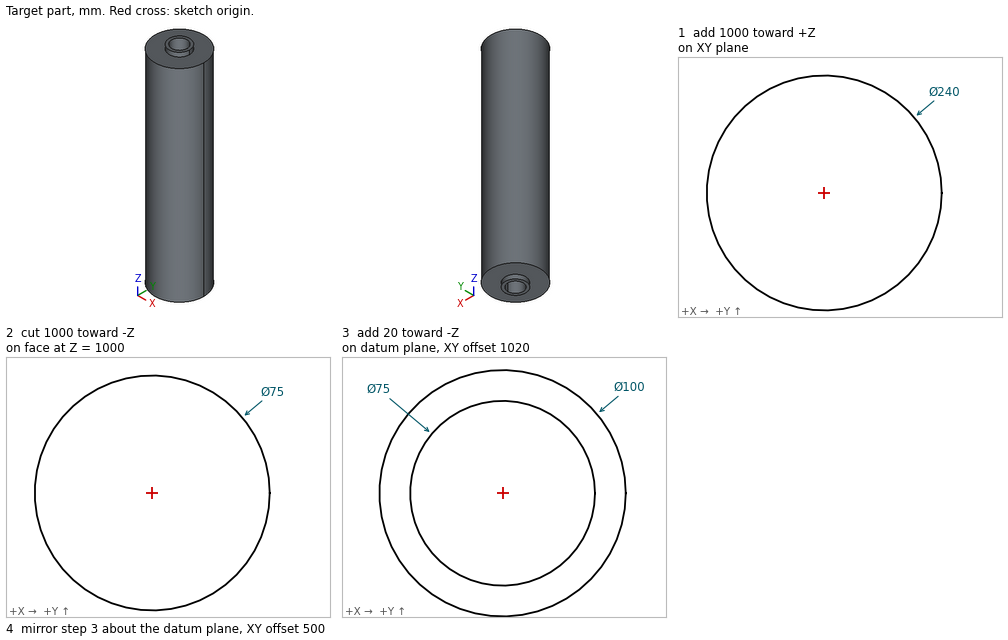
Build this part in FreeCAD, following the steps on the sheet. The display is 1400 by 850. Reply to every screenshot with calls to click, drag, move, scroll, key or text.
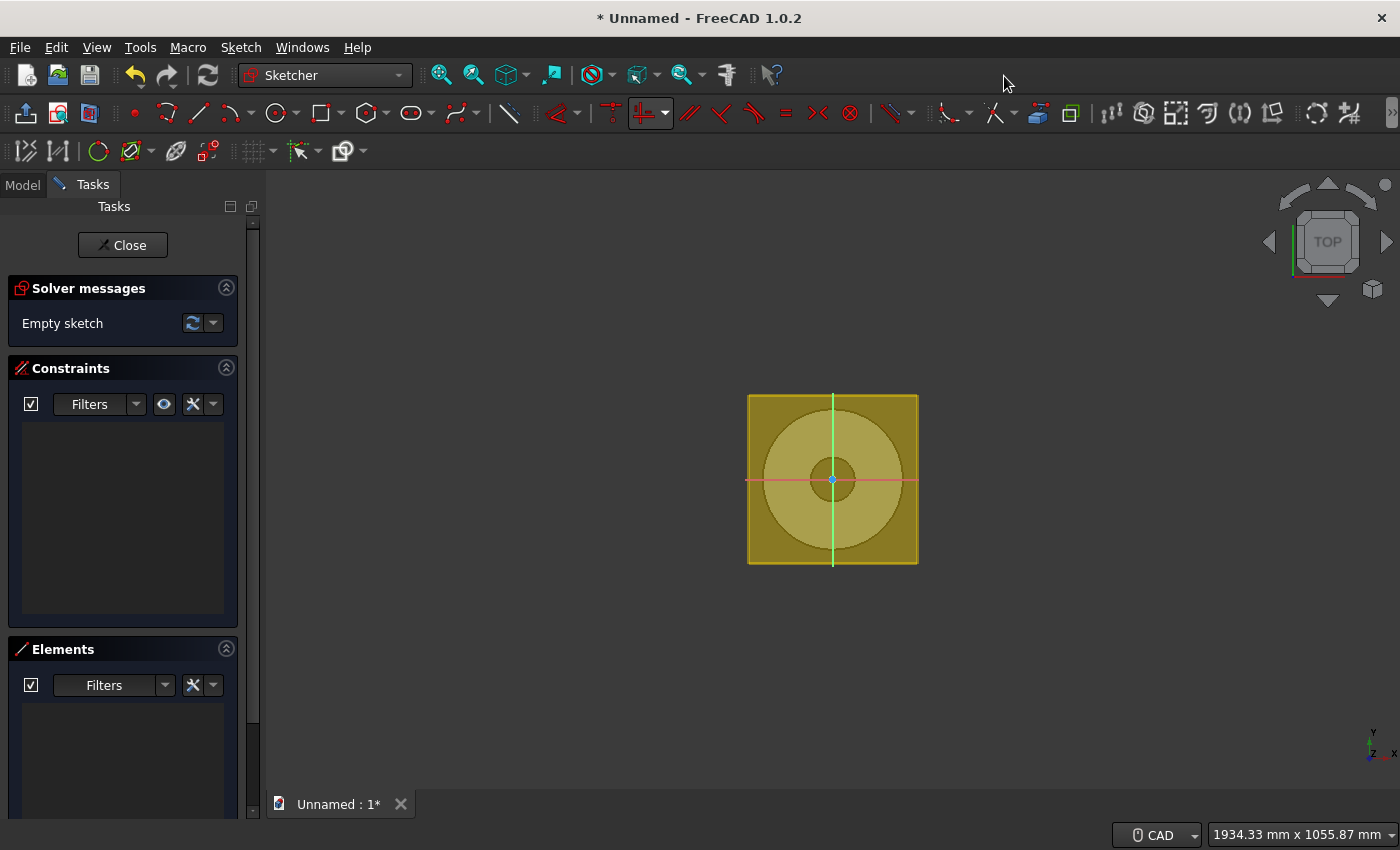
scroll(844, 480, up, 10)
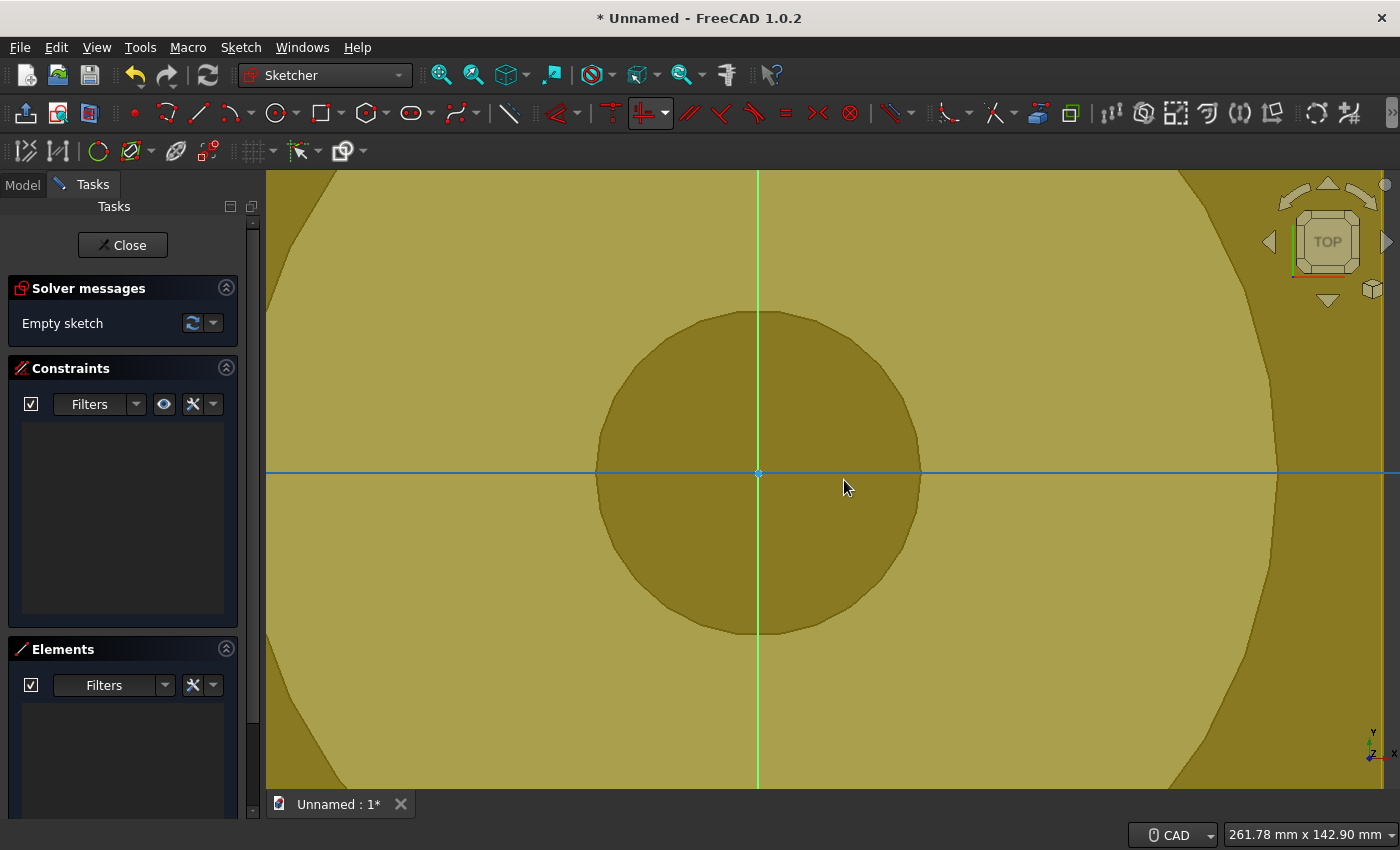
key(g)
key(c)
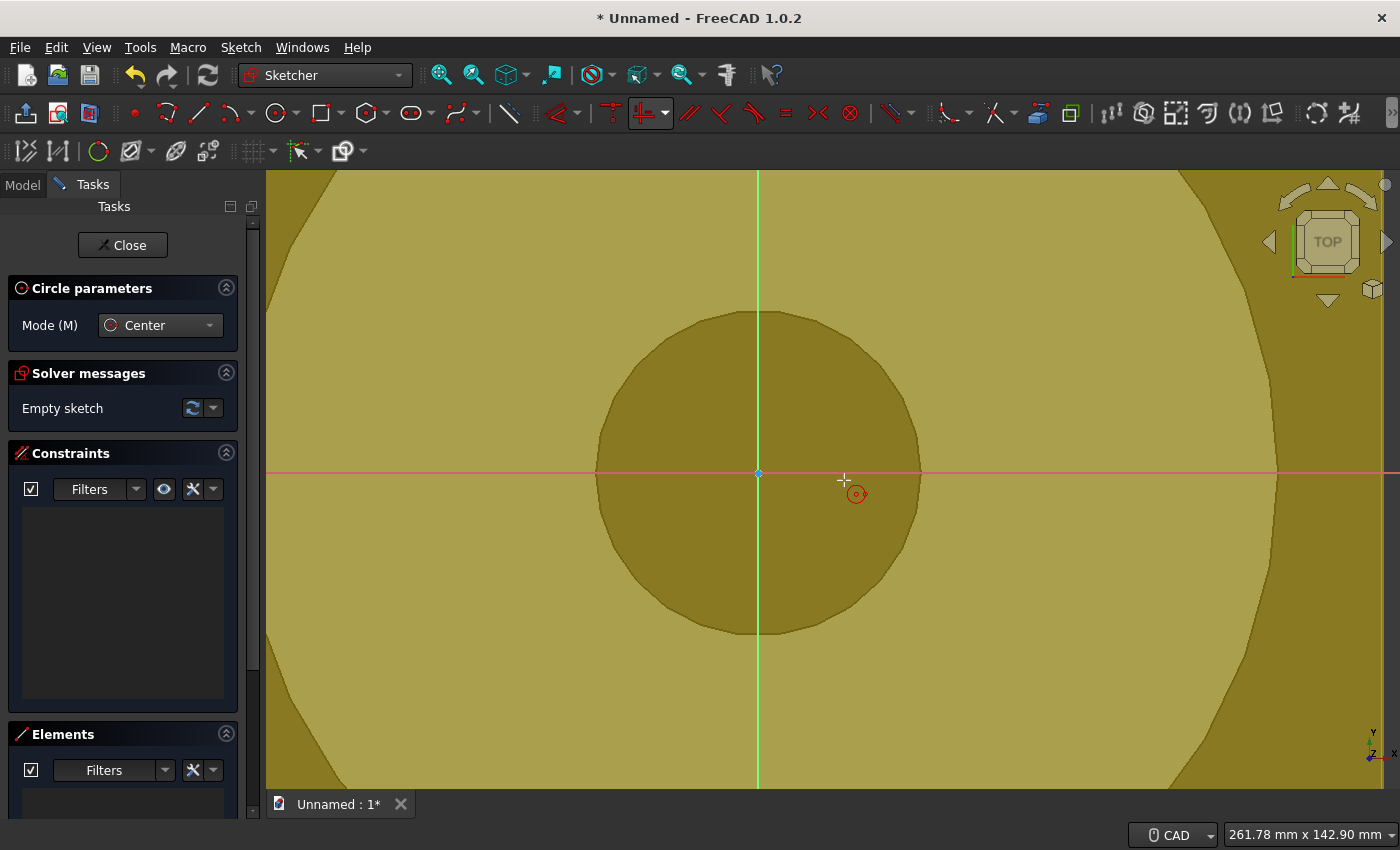
click(758, 473)
click(912, 320)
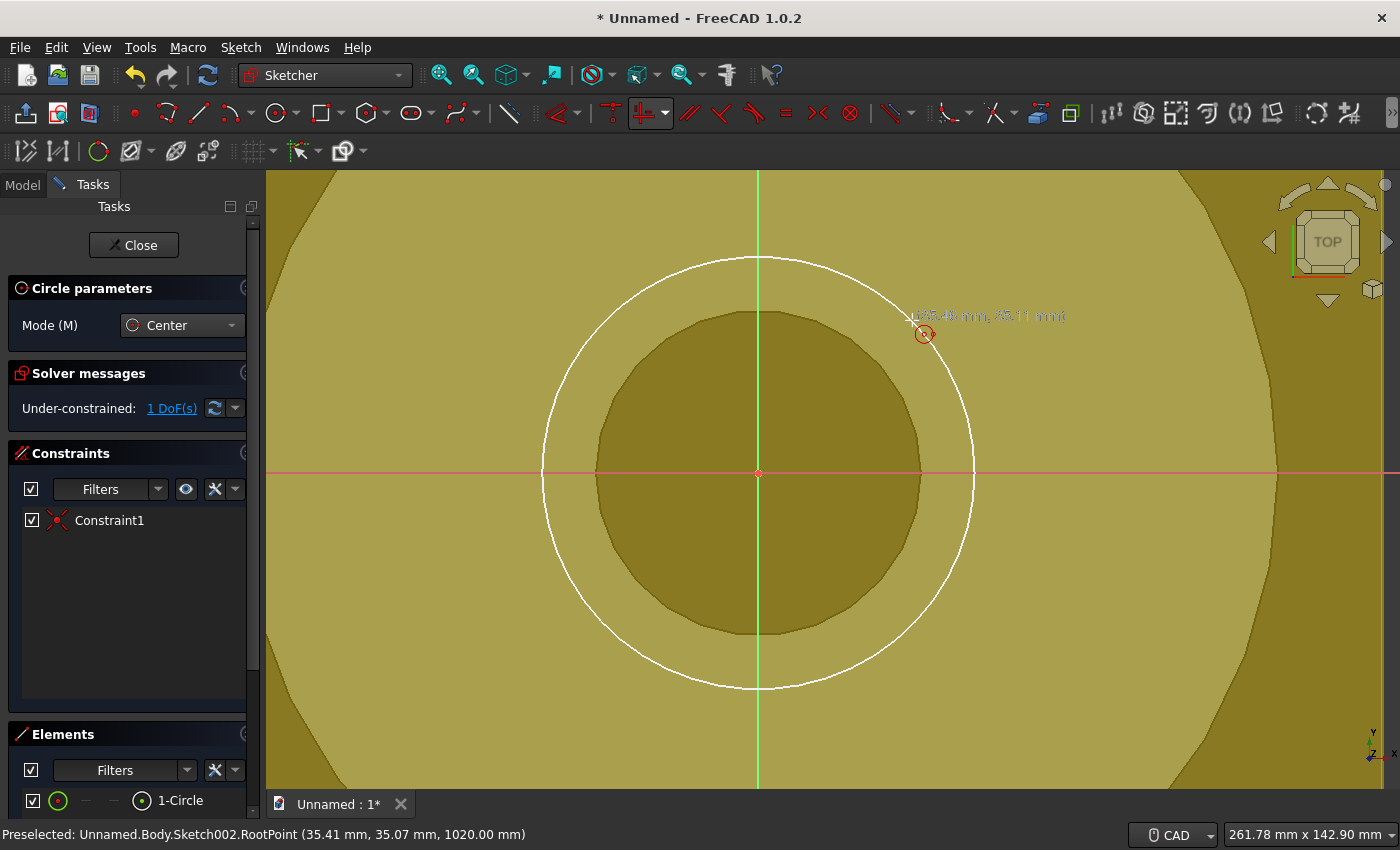
click(758, 473)
click(873, 358)
key(Escape)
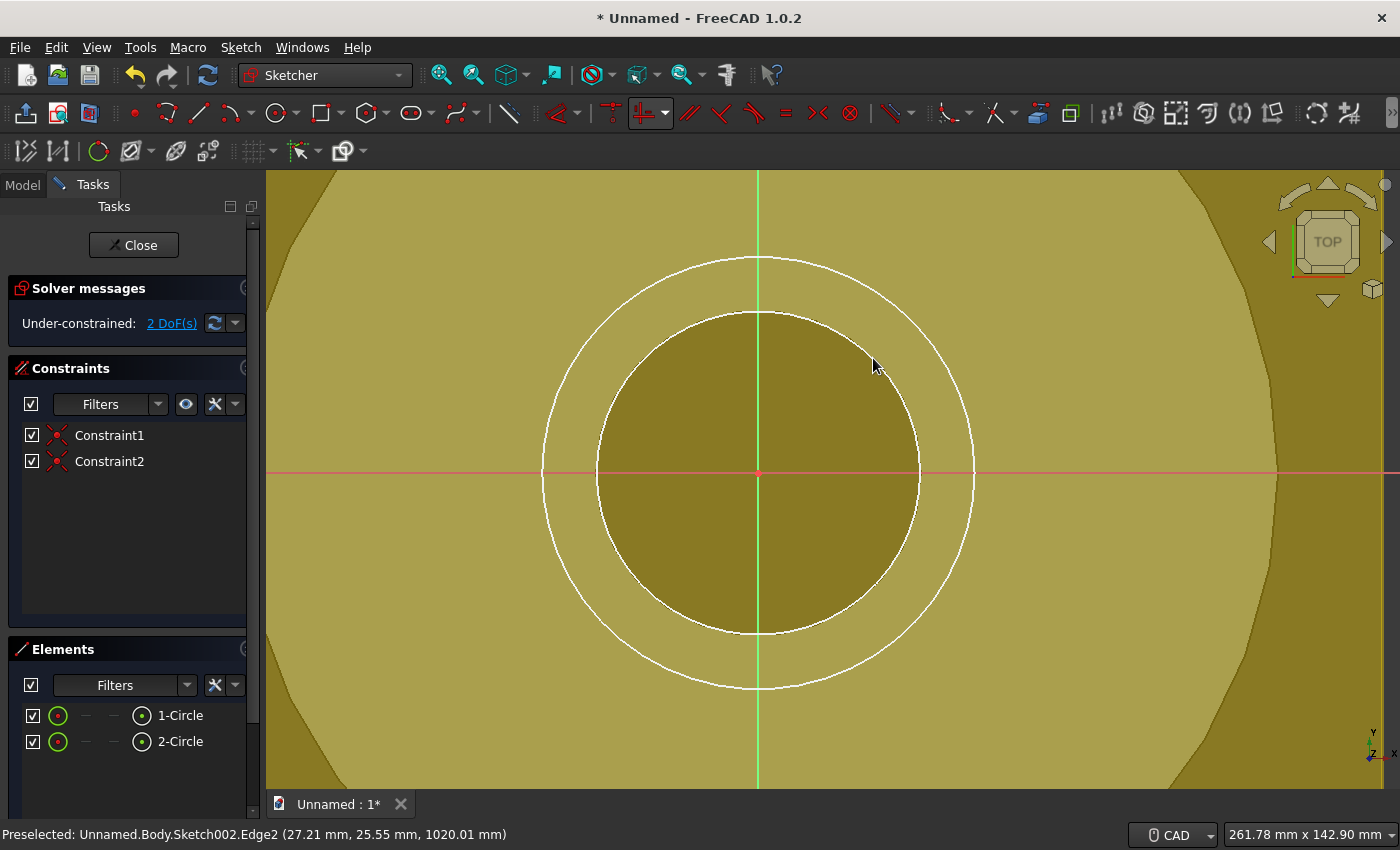
key(d)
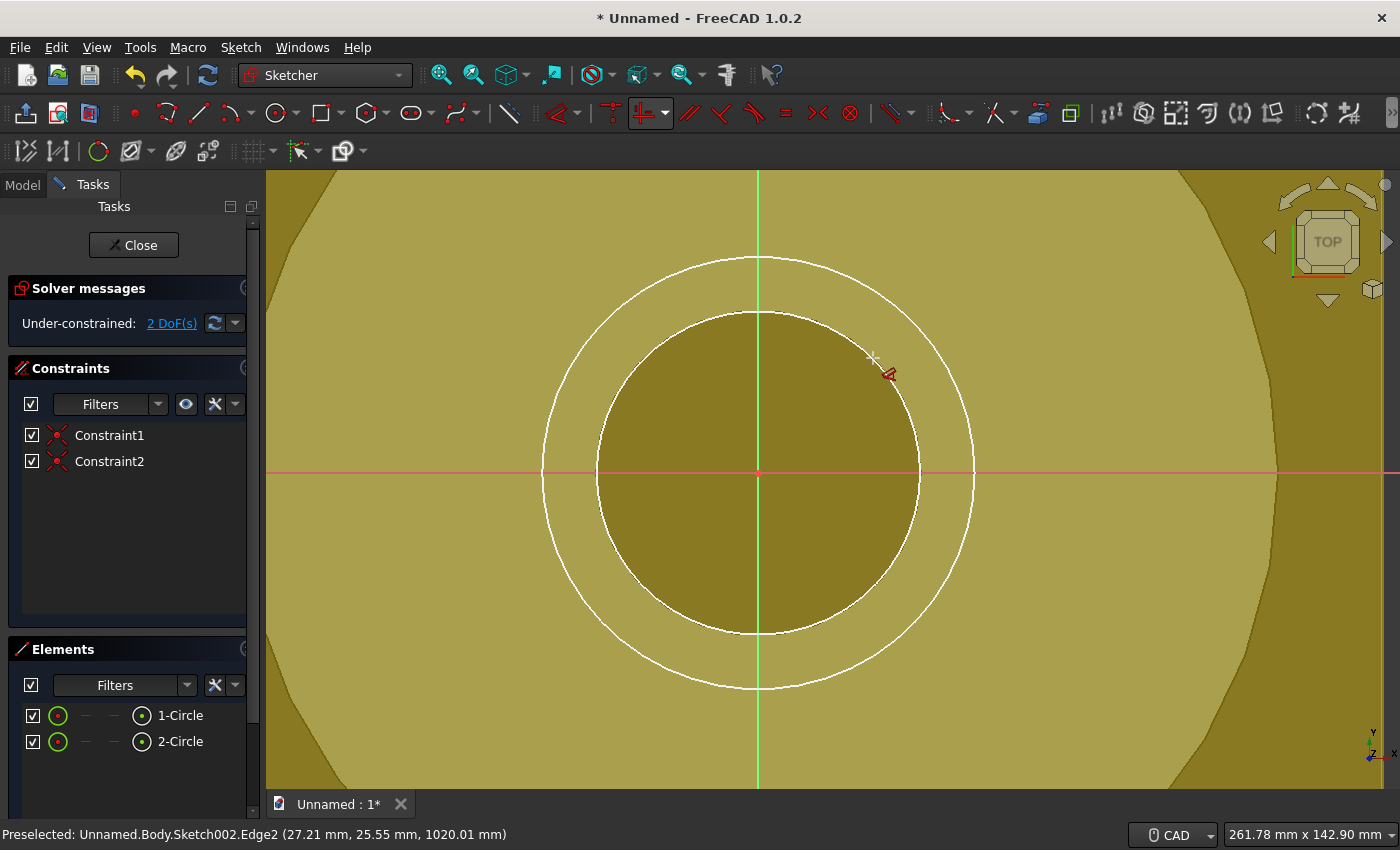
click(911, 320)
click(934, 297)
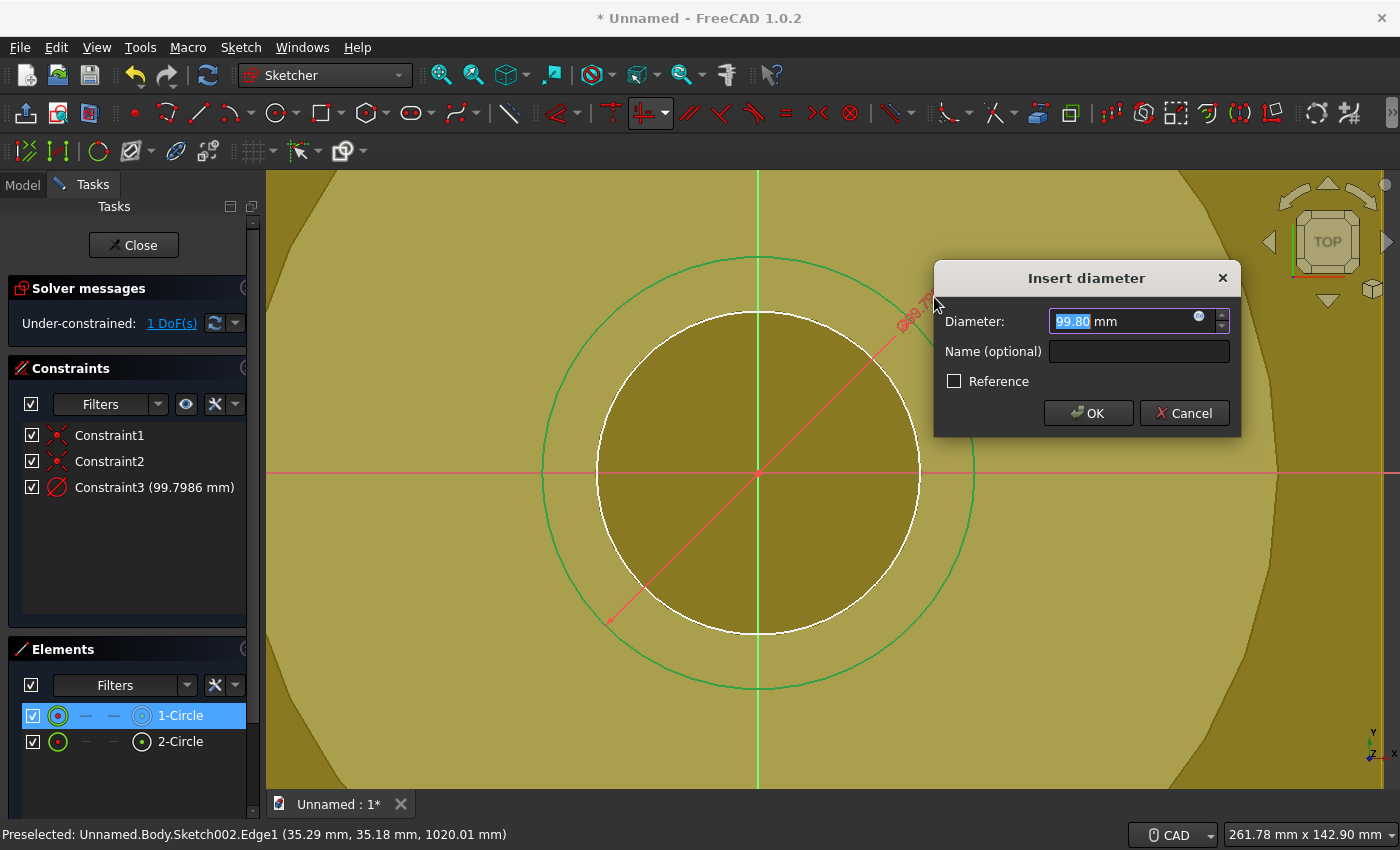
text(100)
key(Return)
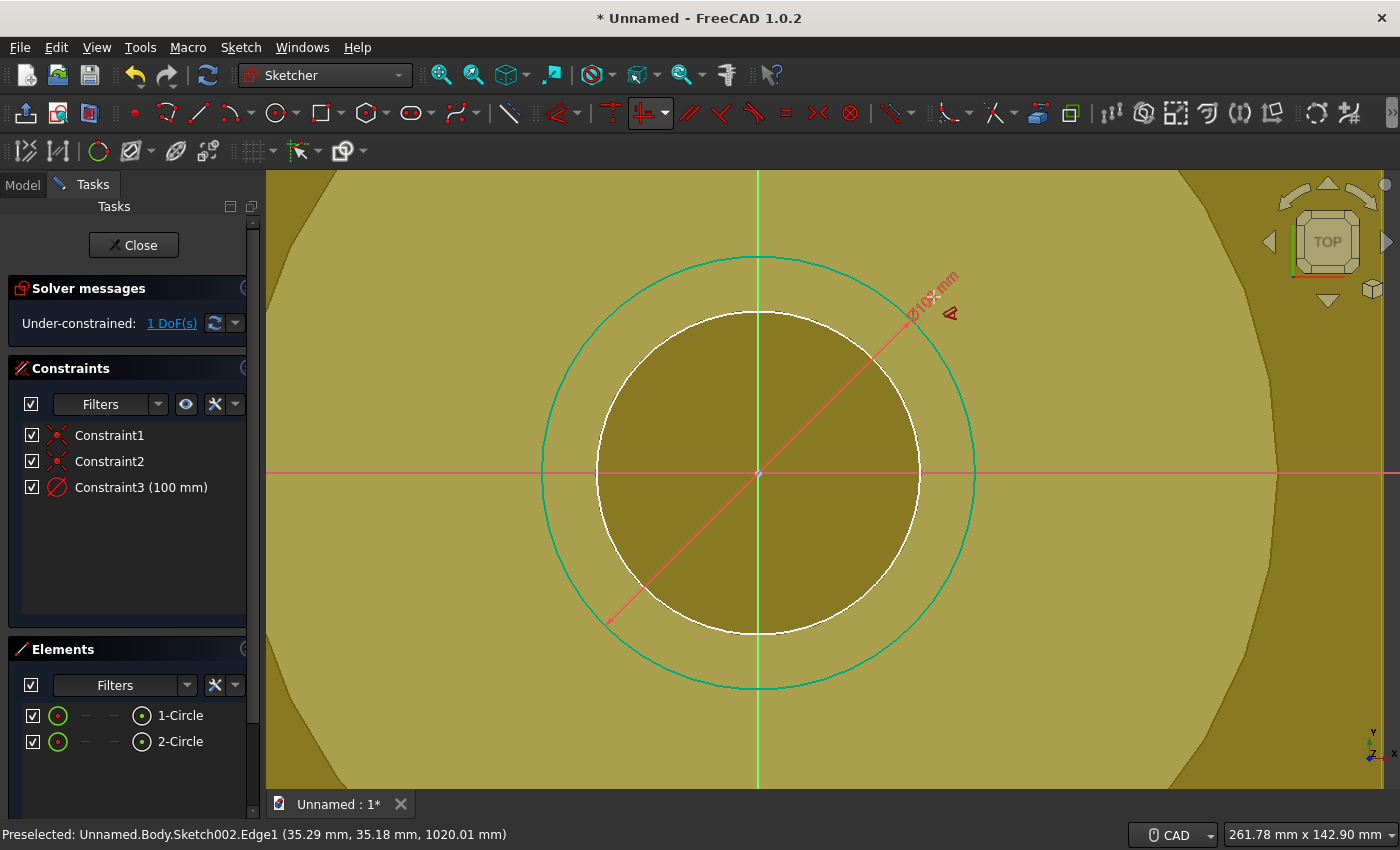
click(872, 358)
click(894, 335)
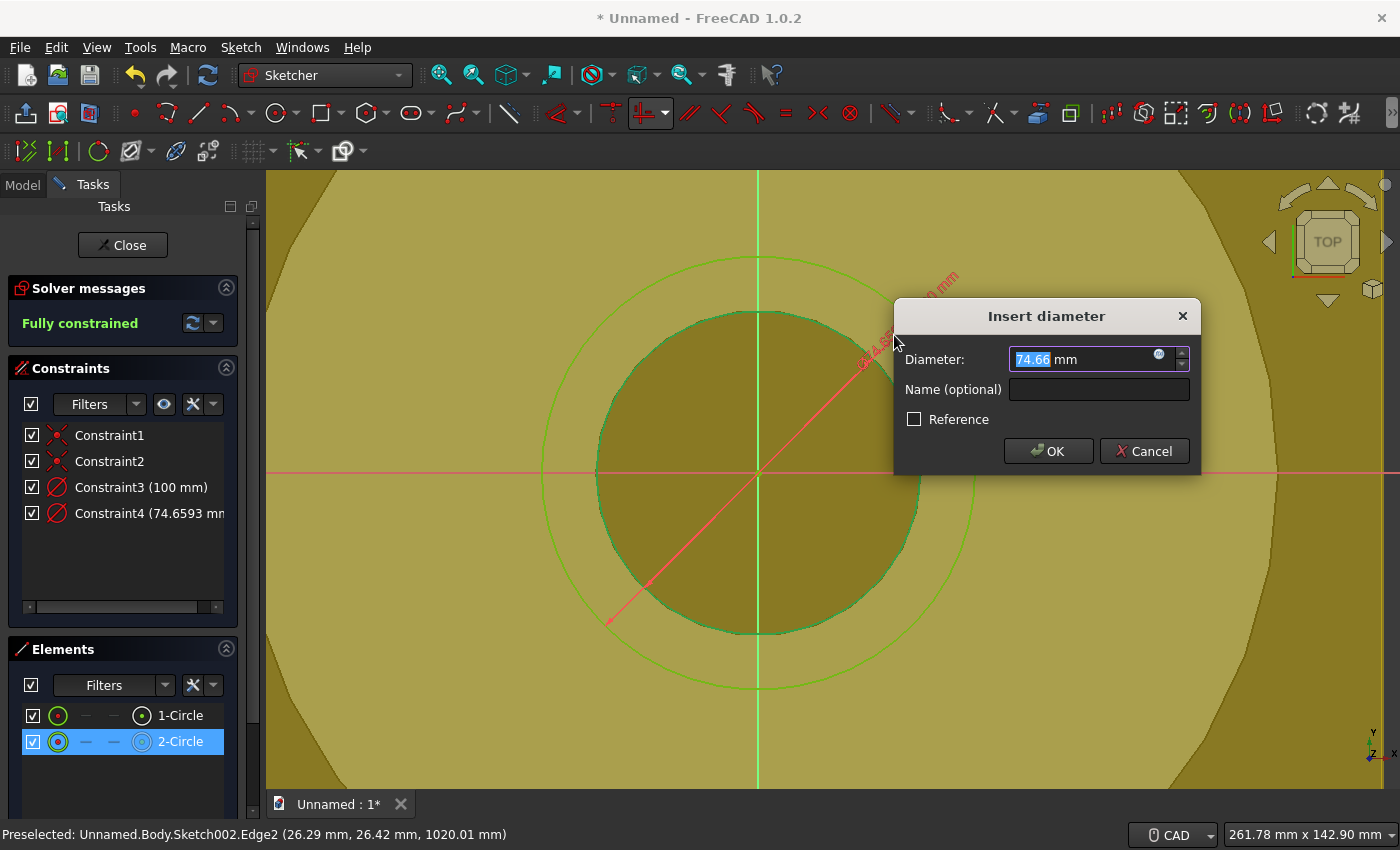
text(75)
key(Return)
key(Escape)